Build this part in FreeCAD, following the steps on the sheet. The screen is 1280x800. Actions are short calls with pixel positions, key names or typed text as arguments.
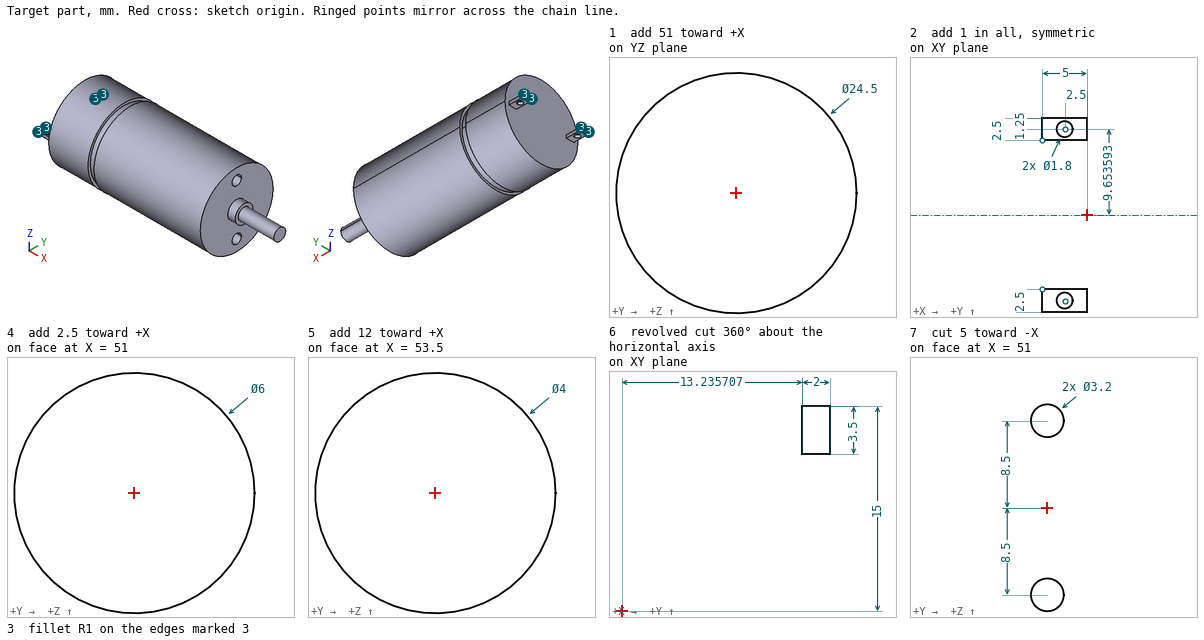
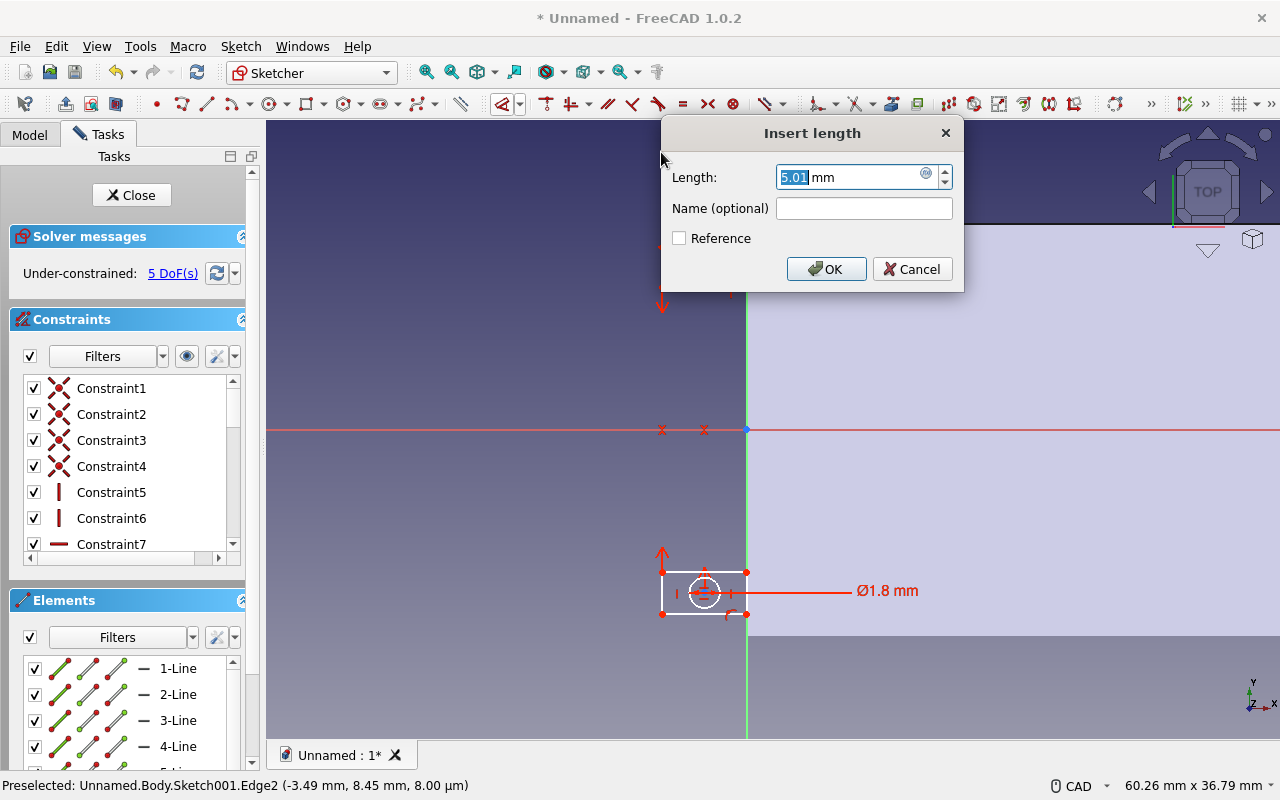
text(5)
key(Return)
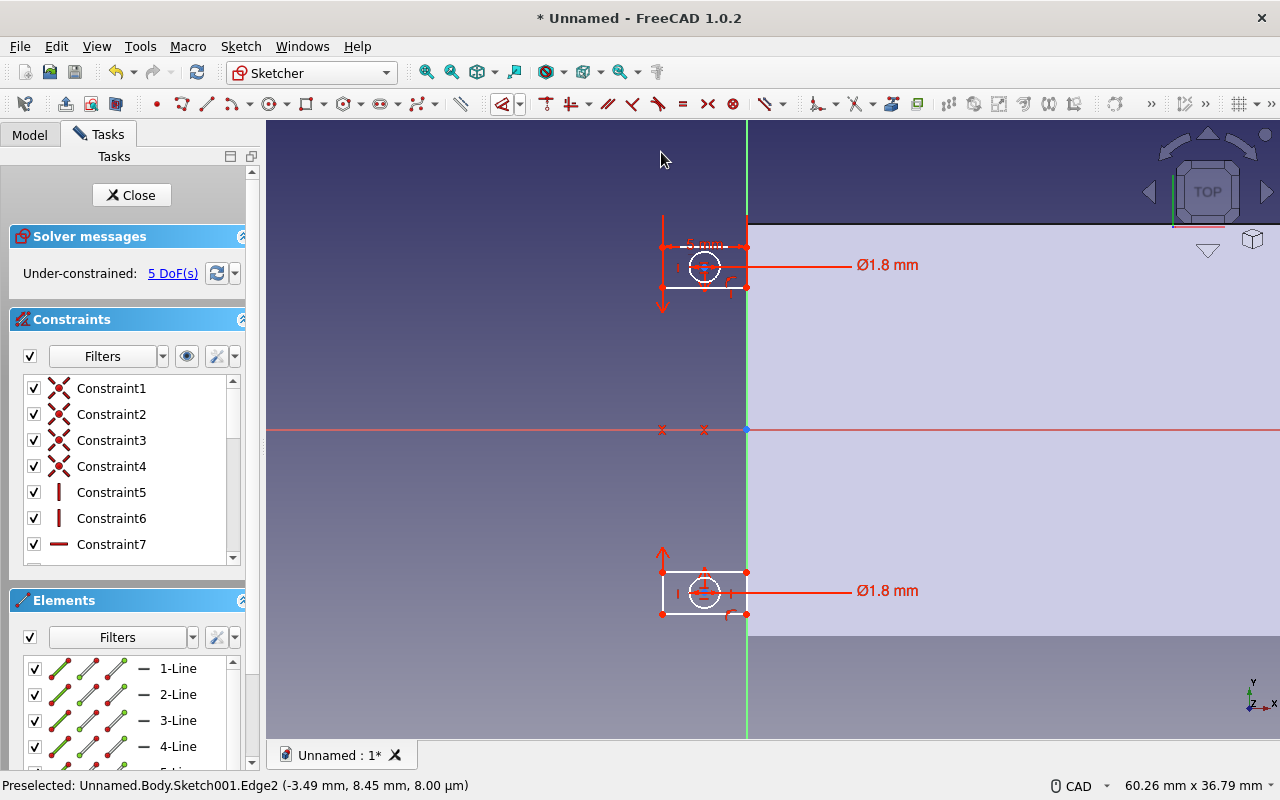
click(663, 260)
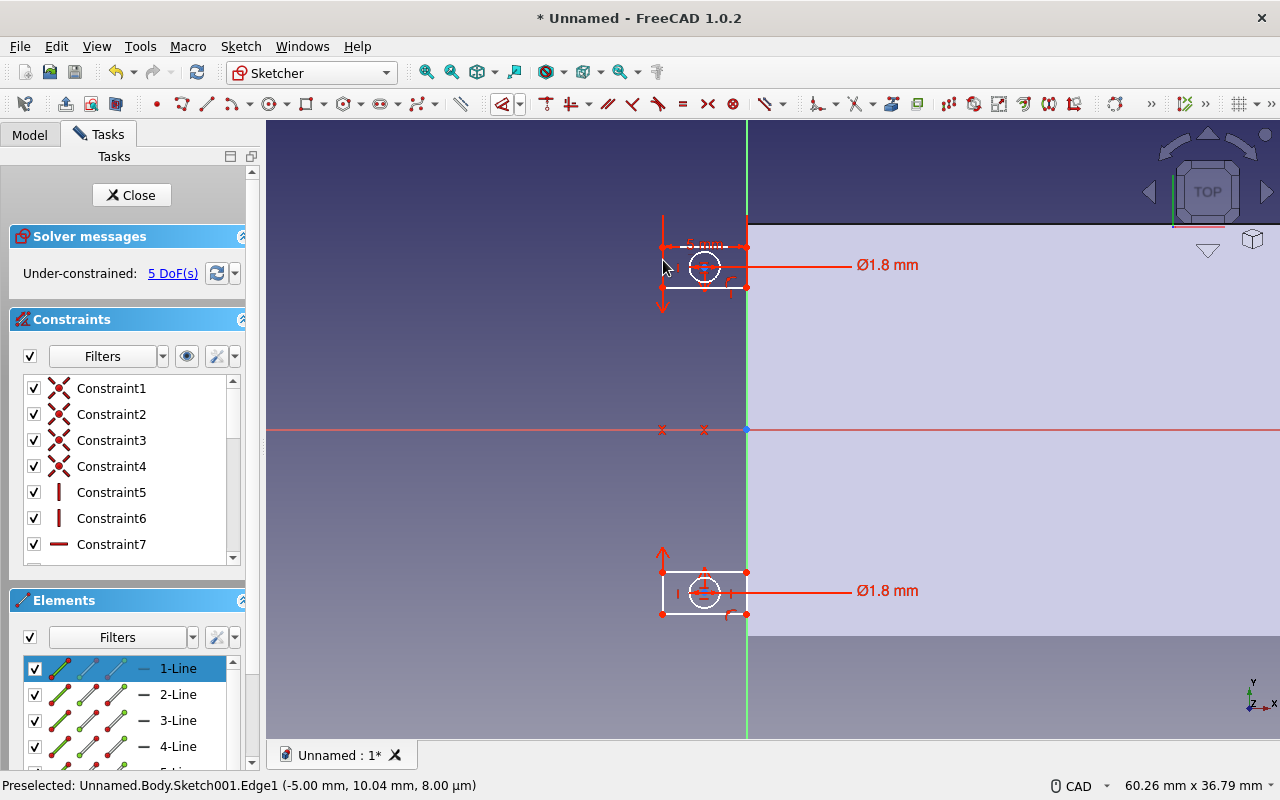
click(520, 104)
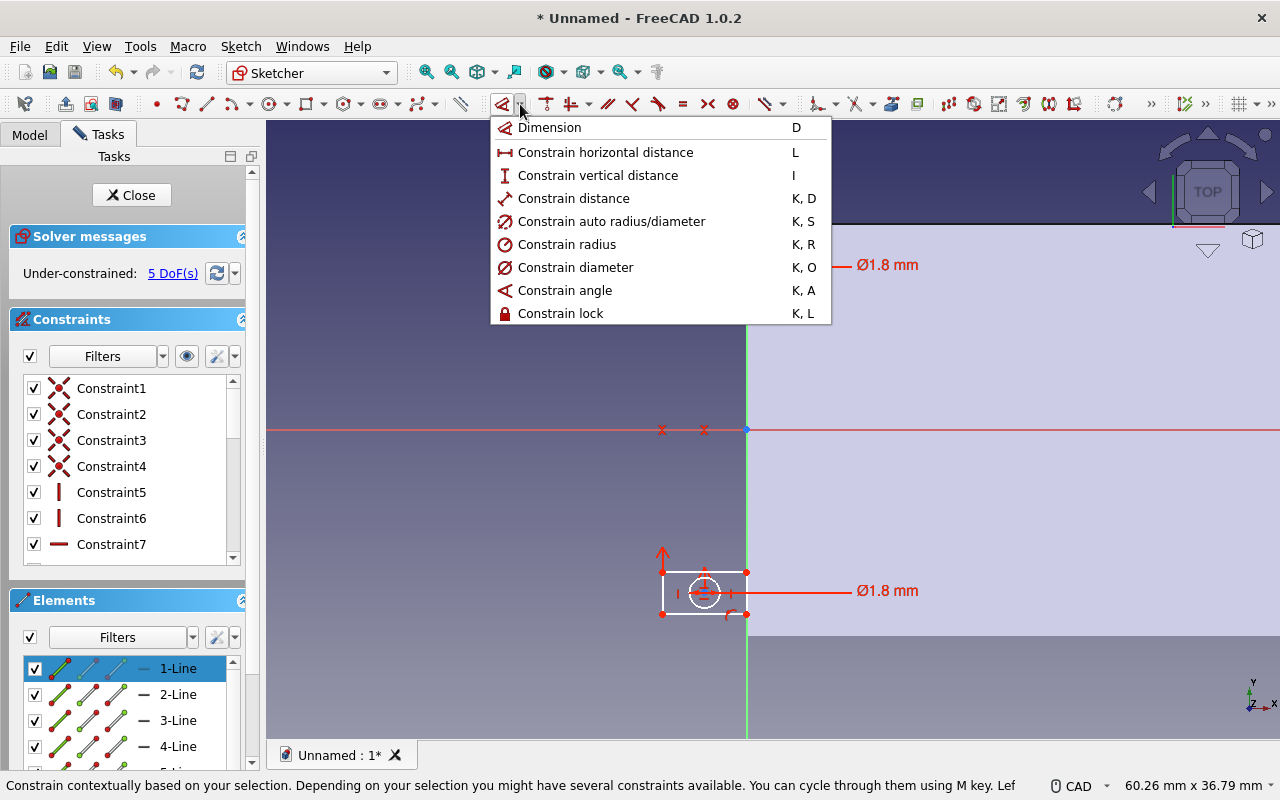
click(661, 176)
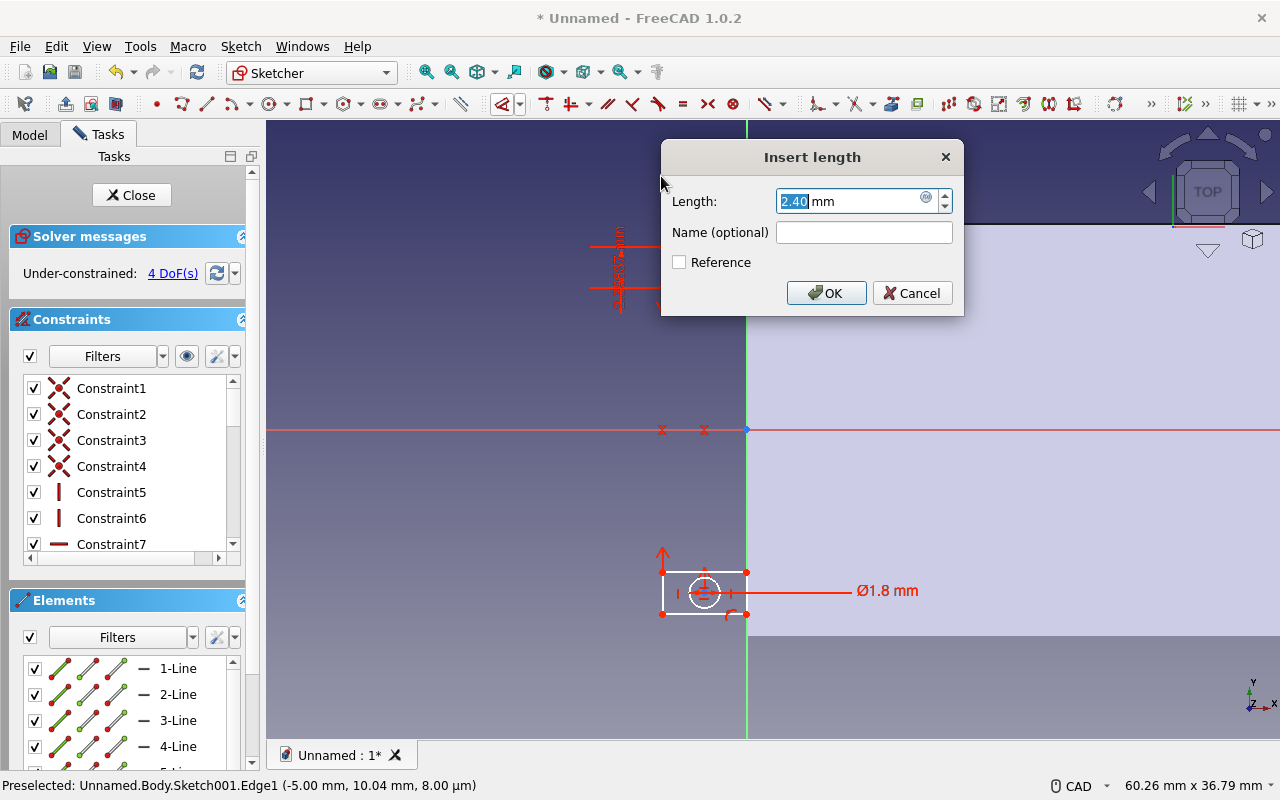
text(2.5)
key(Return)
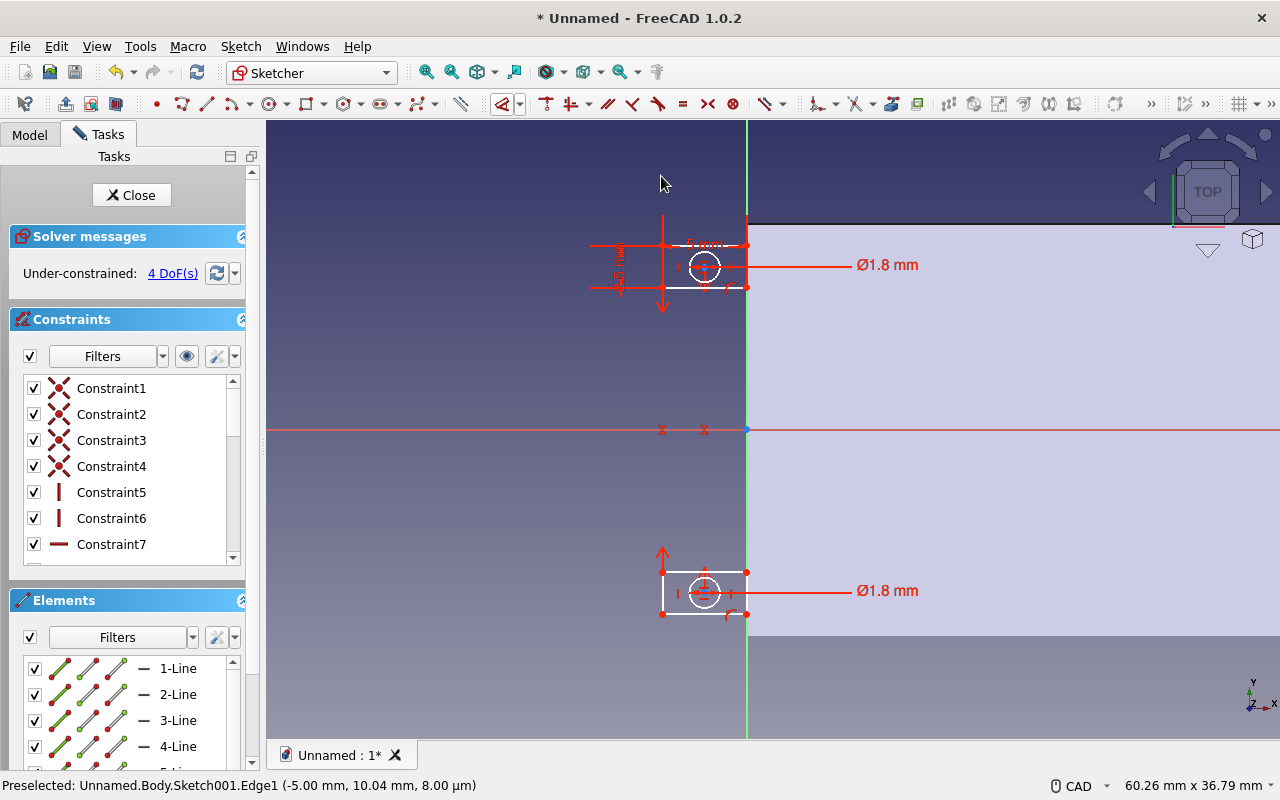
click(663, 585)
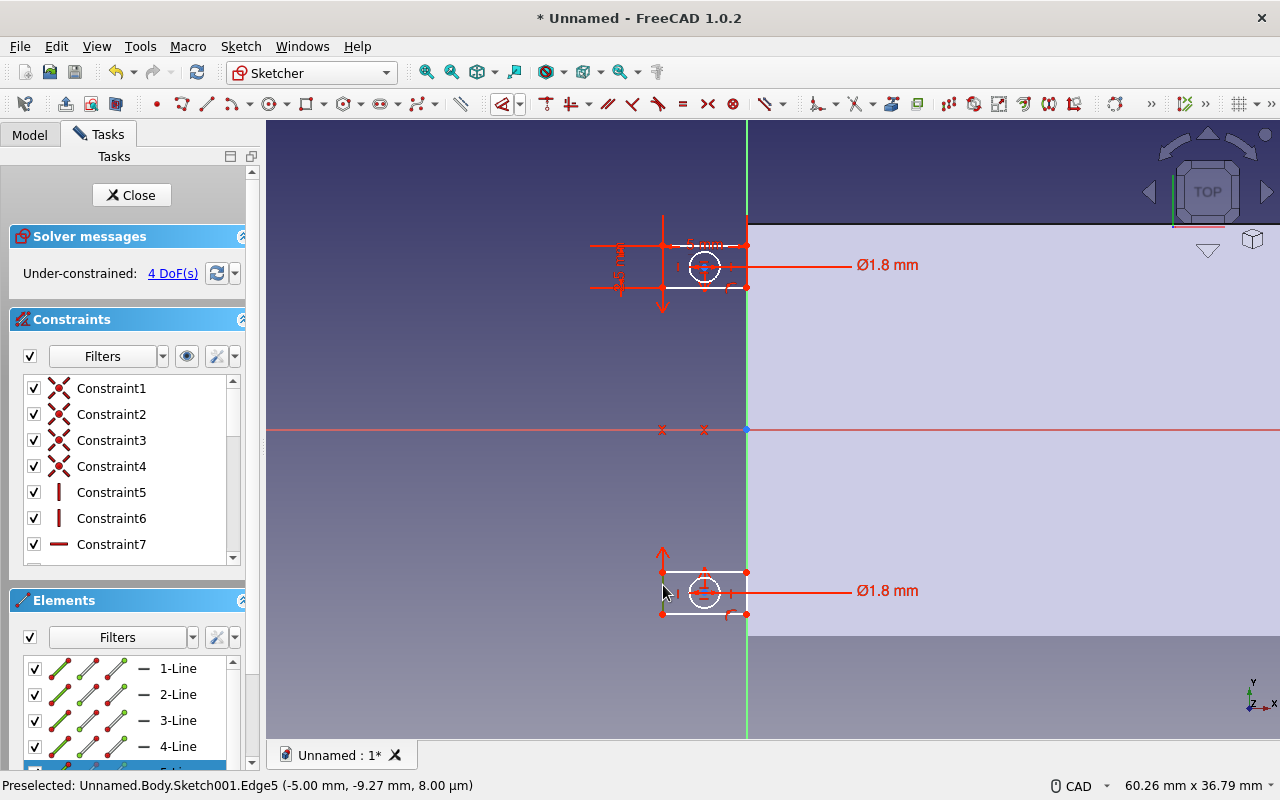
click(520, 104)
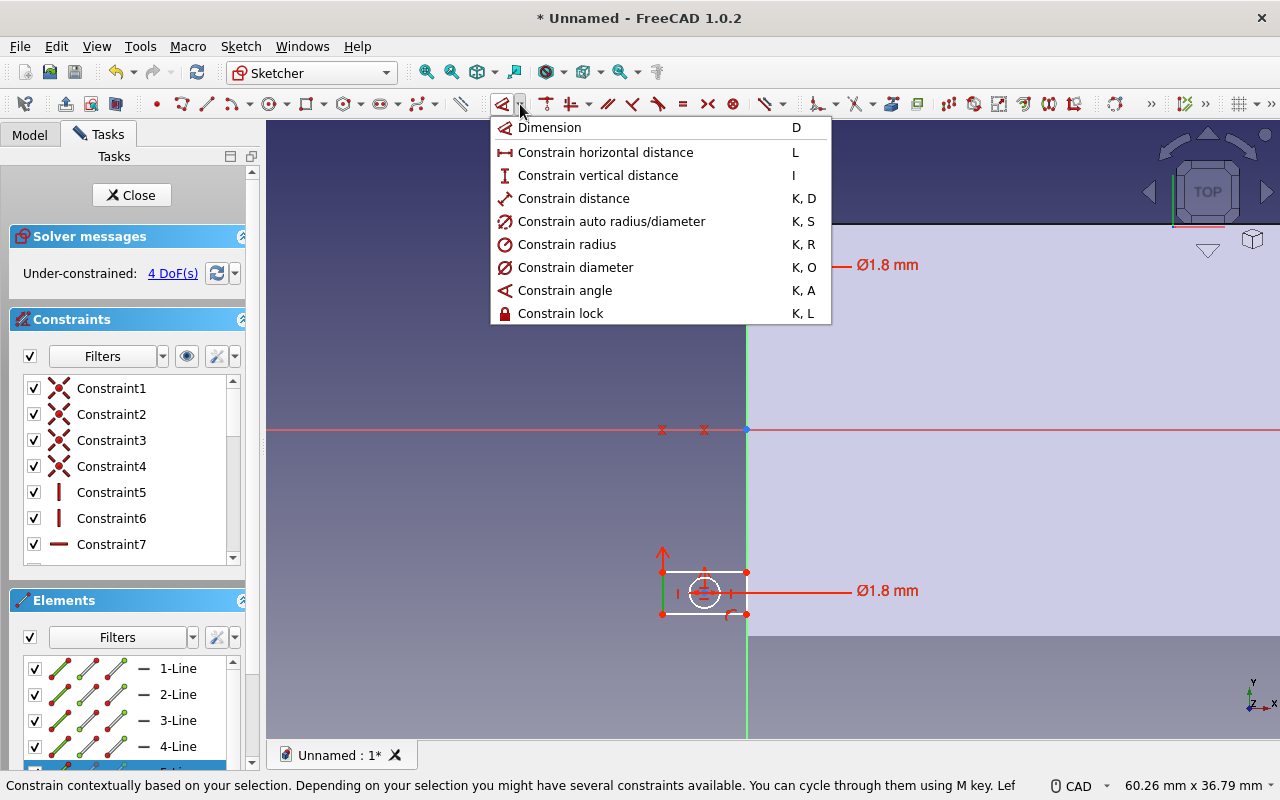
click(661, 176)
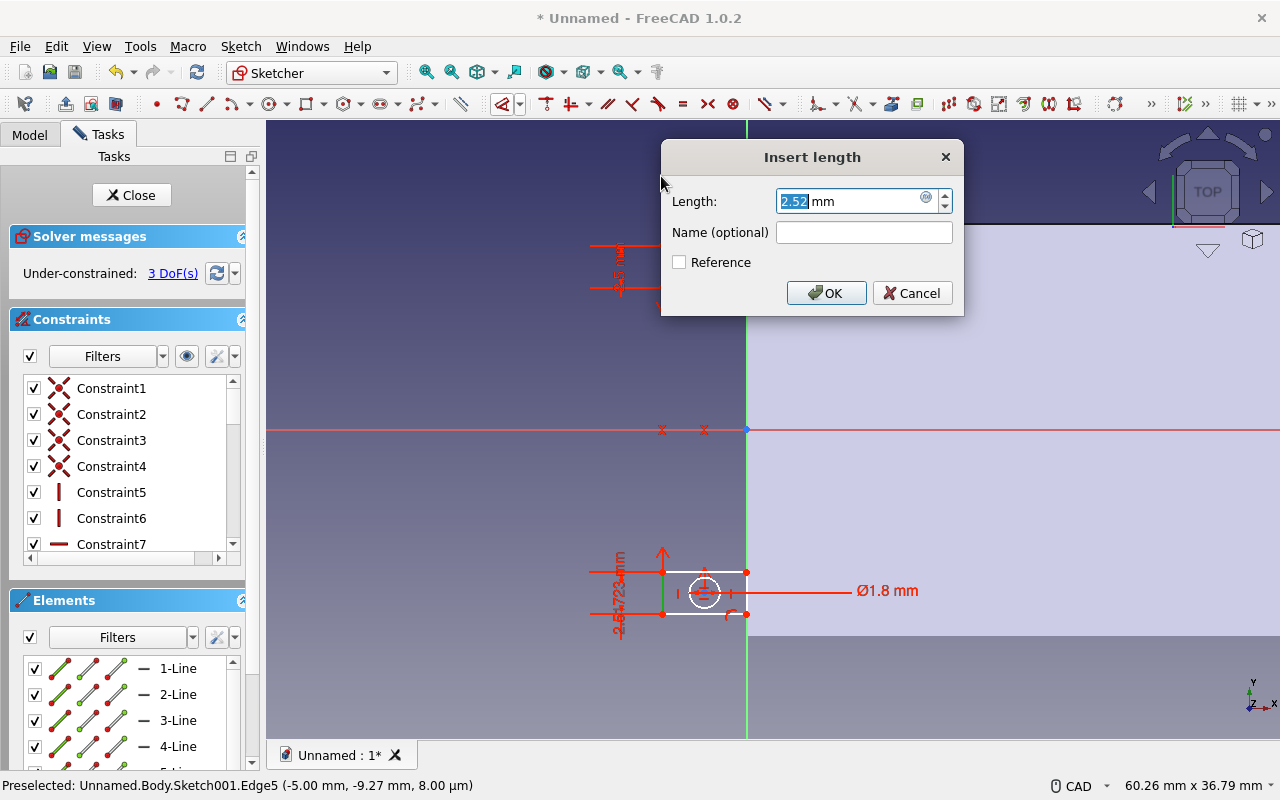
text(2.5)
key(Return)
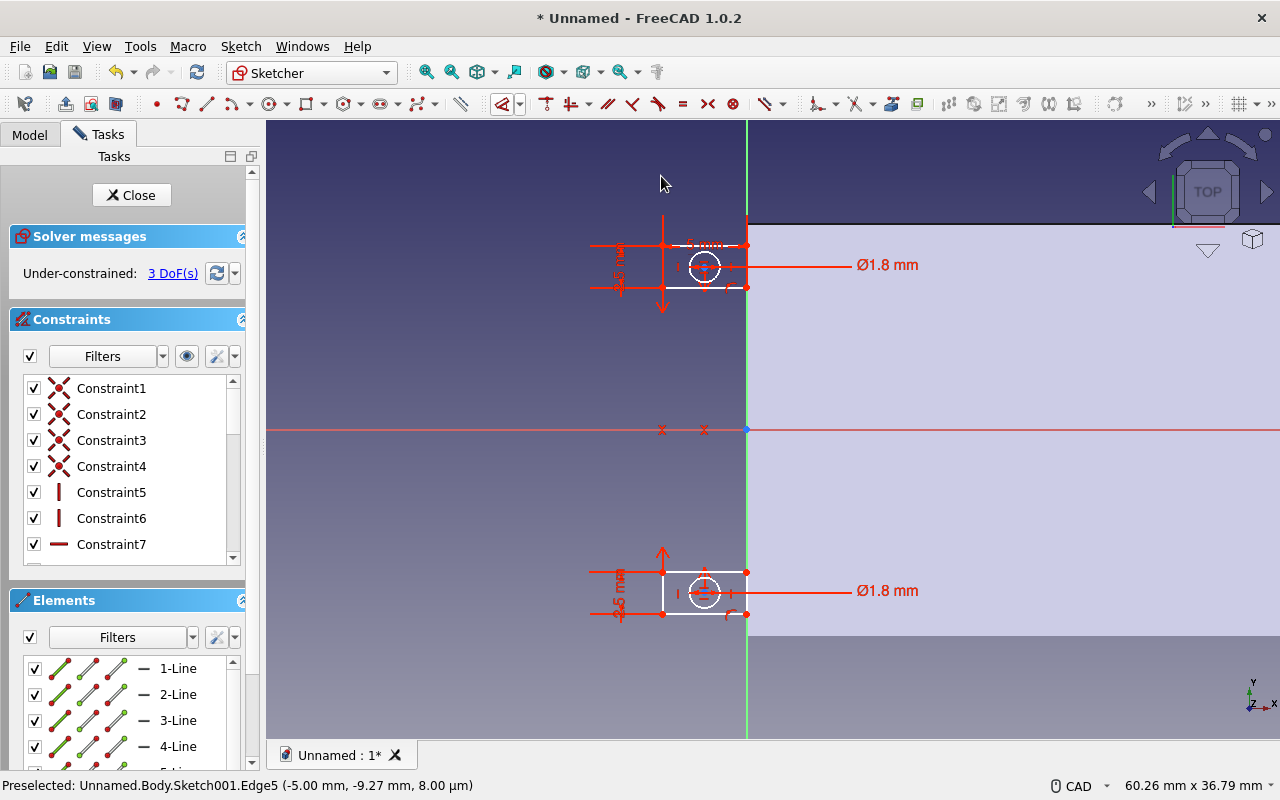
click(705, 267)